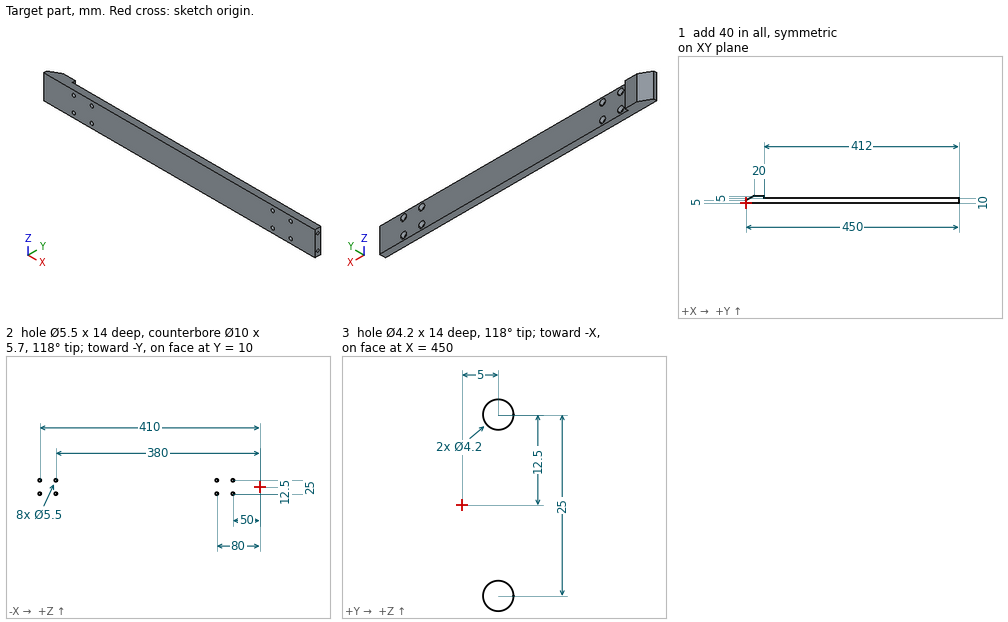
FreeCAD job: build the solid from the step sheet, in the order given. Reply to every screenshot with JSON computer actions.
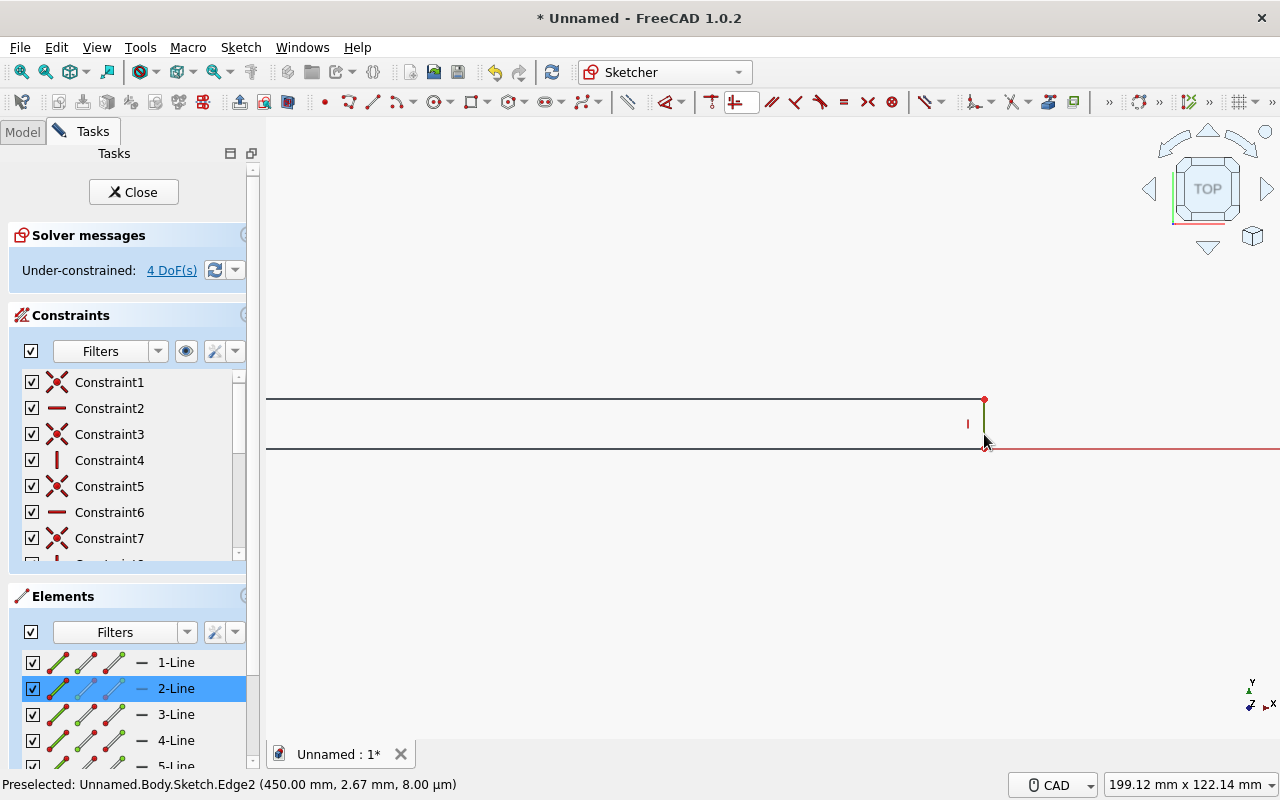
{"action": "left_click", "coordinate": [684, 102]}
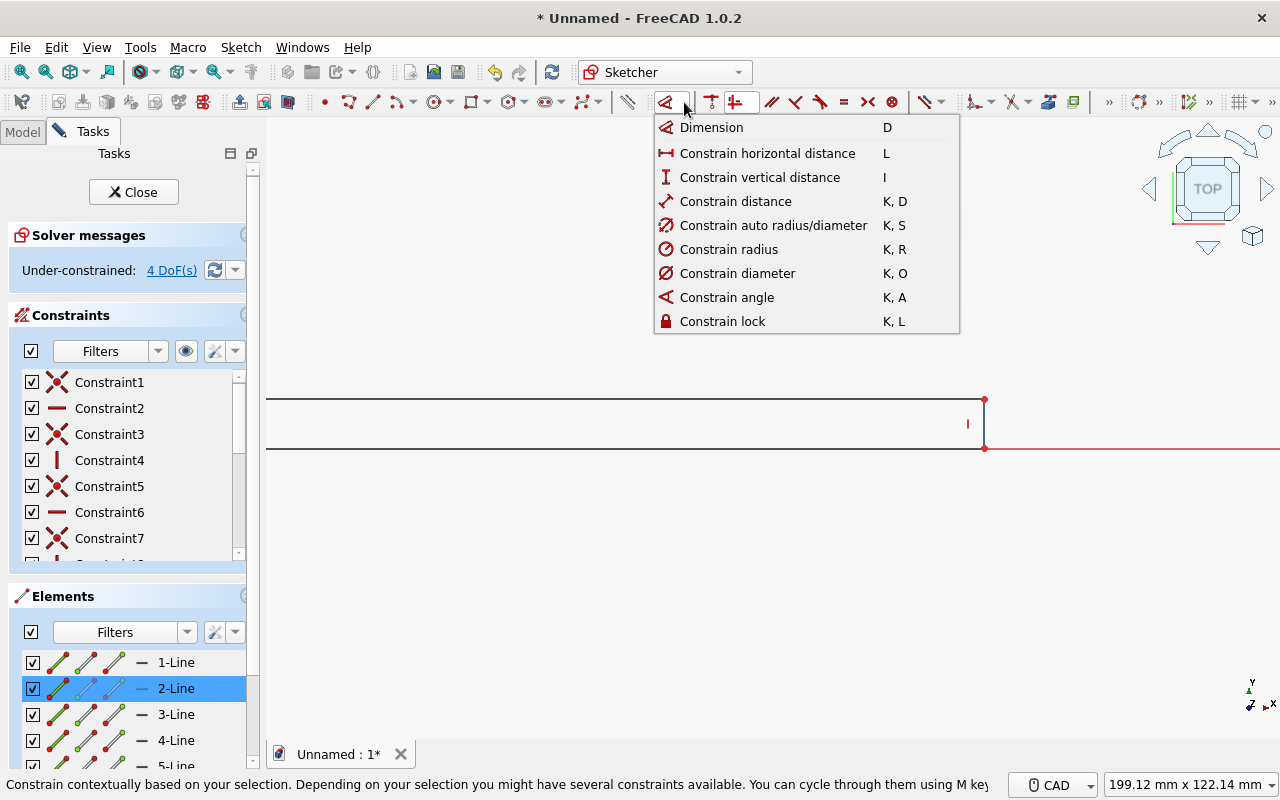
{"action": "left_click", "coordinate": [807, 177]}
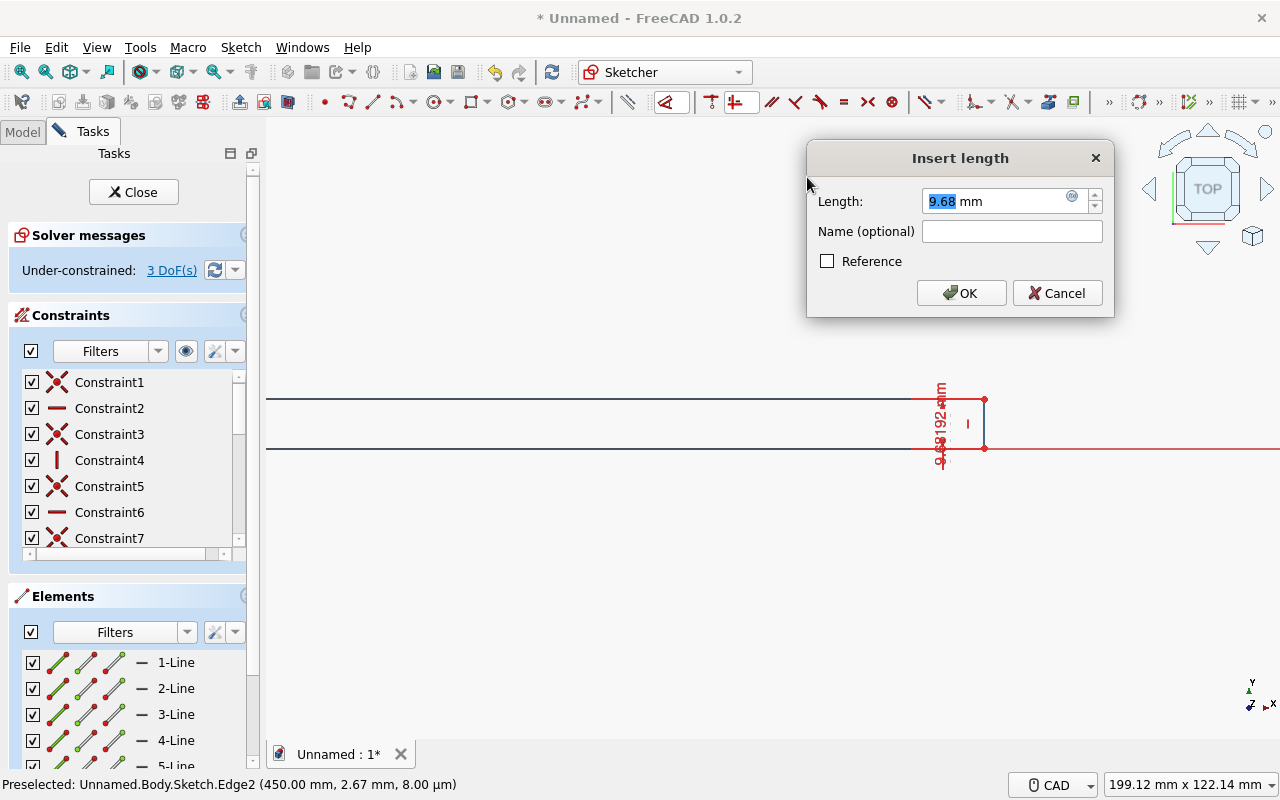
{"action": "type", "text": "10"}
{"action": "key", "text": "Return"}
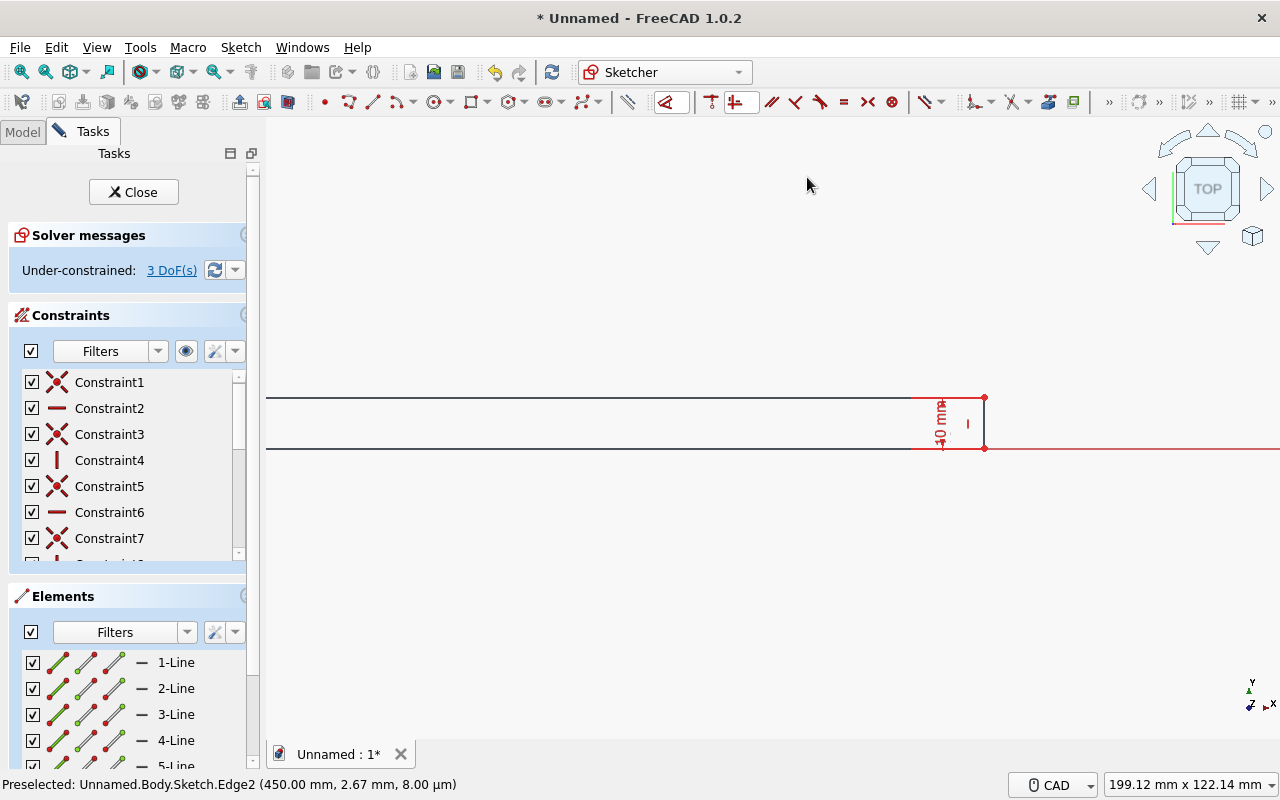
{"action": "scroll", "coordinate": [988, 434], "scroll_direction": "down", "scroll_amount": 7}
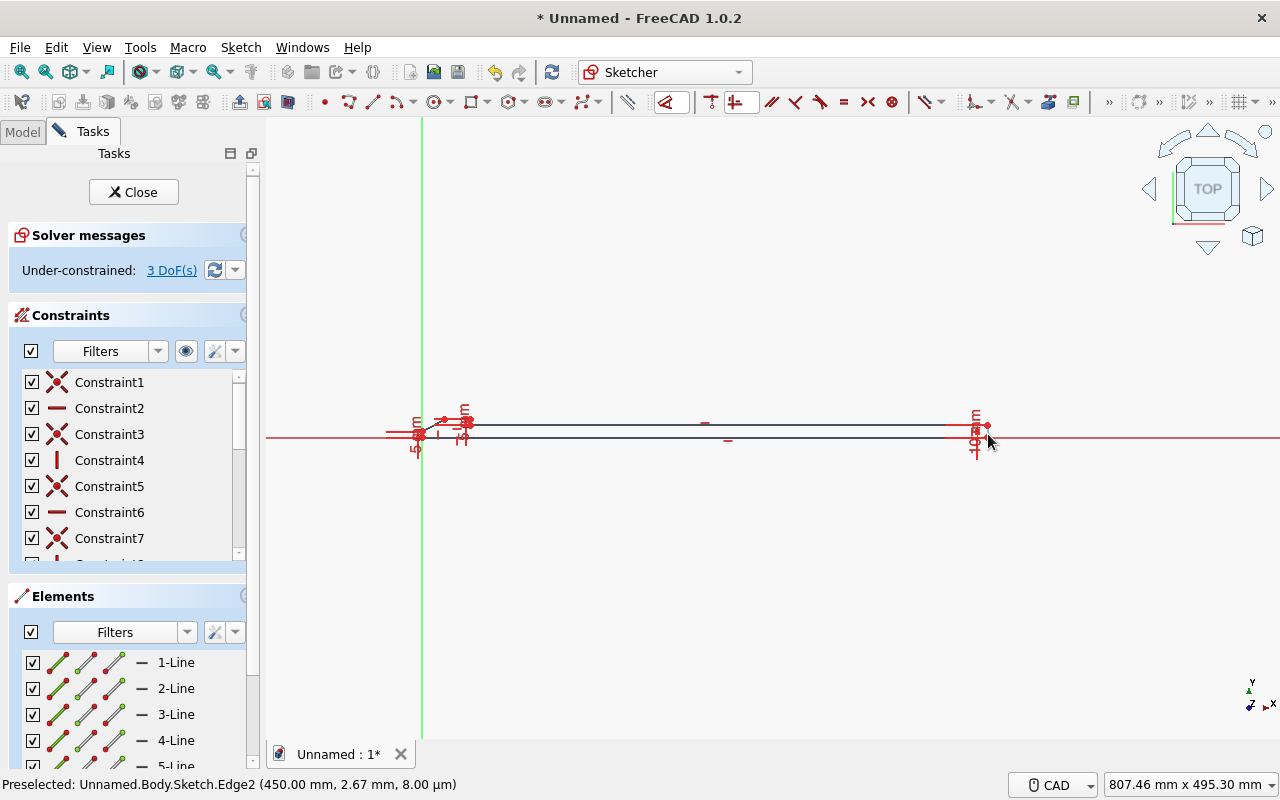
{"action": "scroll", "coordinate": [463, 419], "scroll_direction": "up", "scroll_amount": 3}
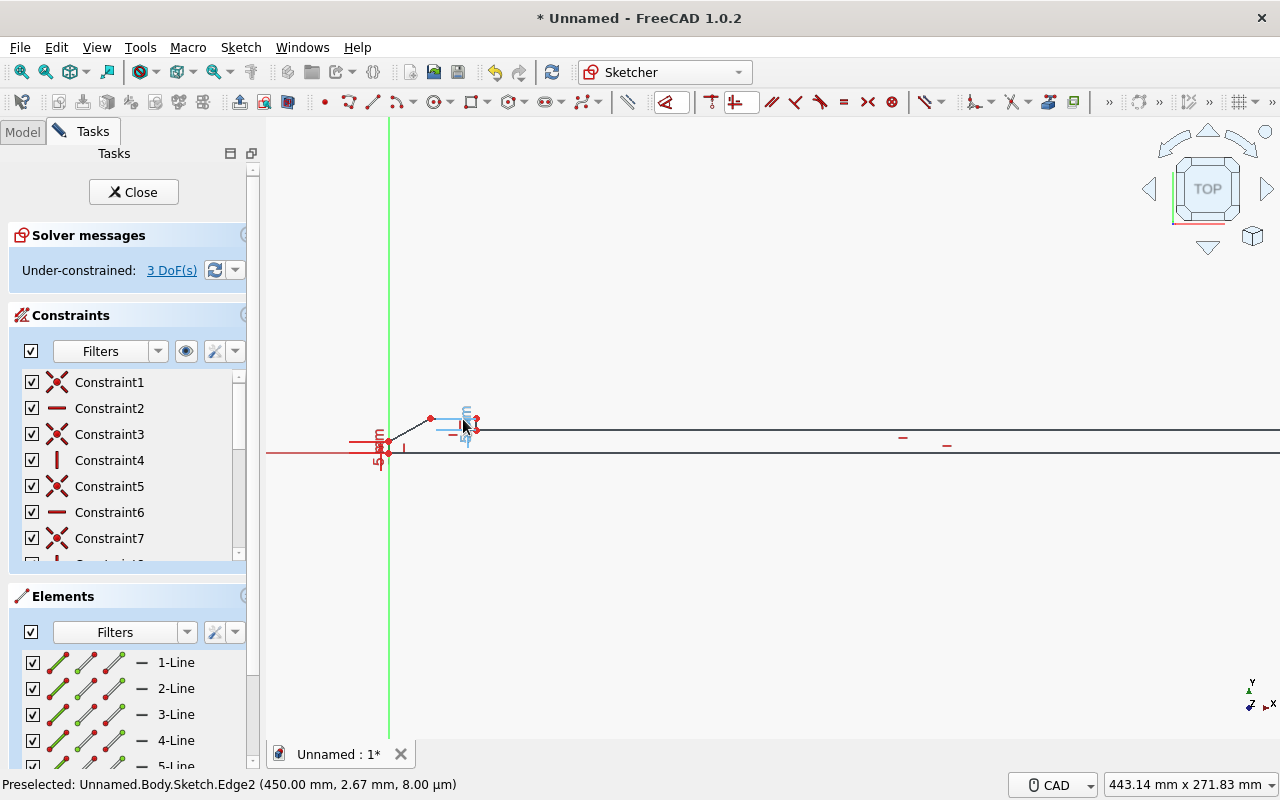
{"action": "left_click", "coordinate": [444, 419]}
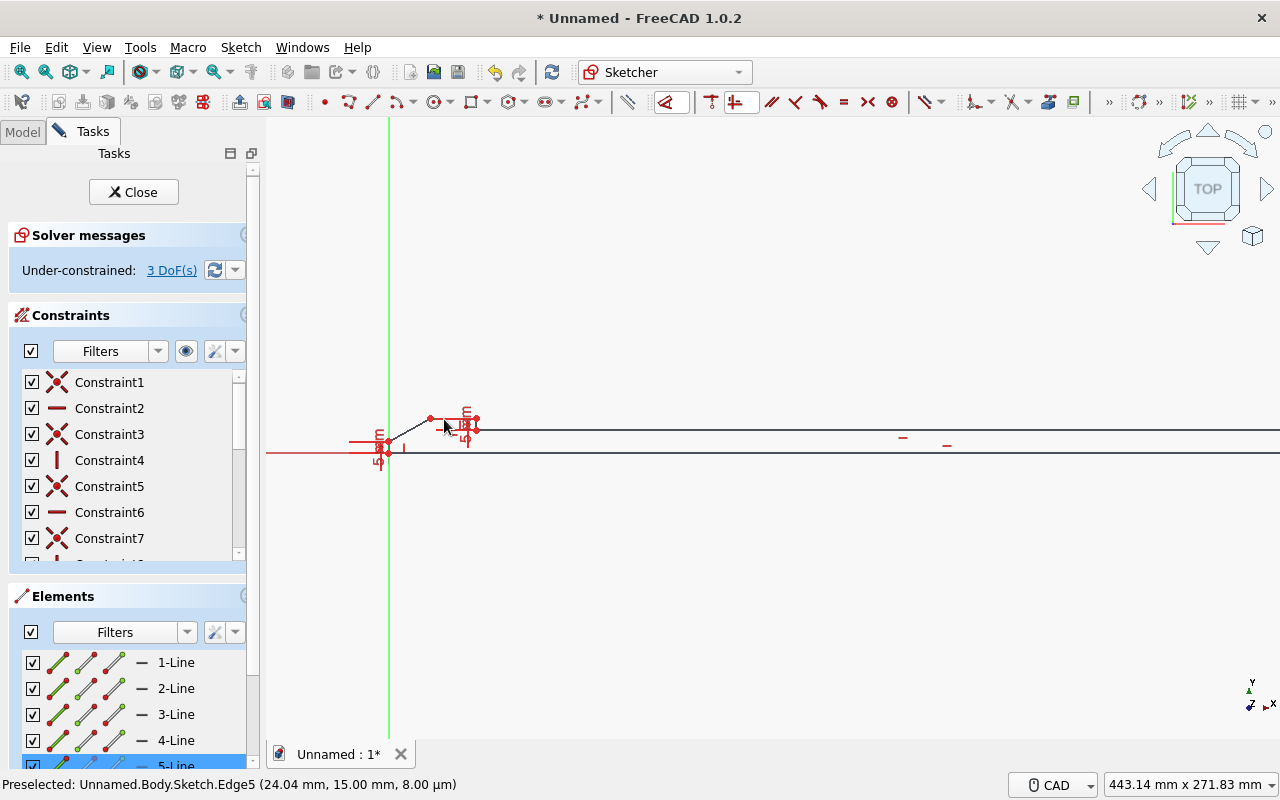
{"action": "key", "text": "l"}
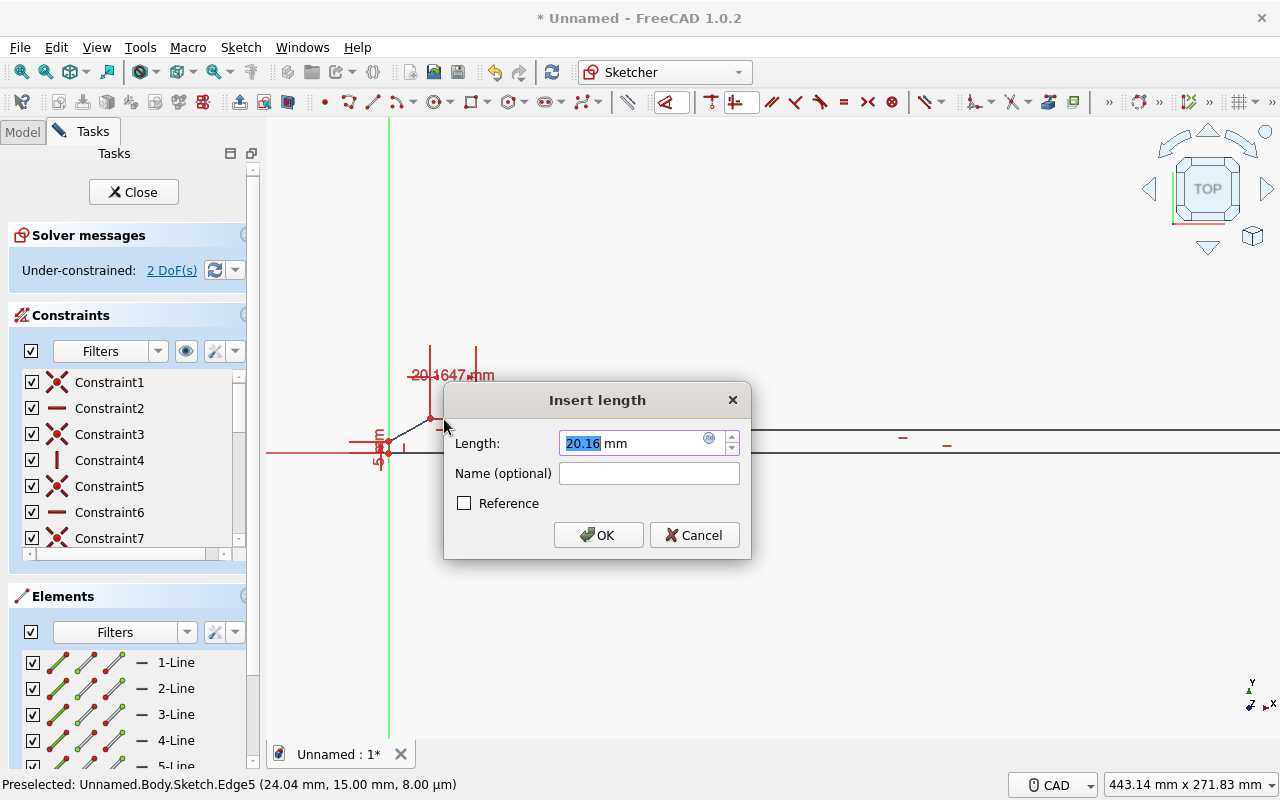
{"action": "type", "text": "20"}
{"action": "key", "text": "Return"}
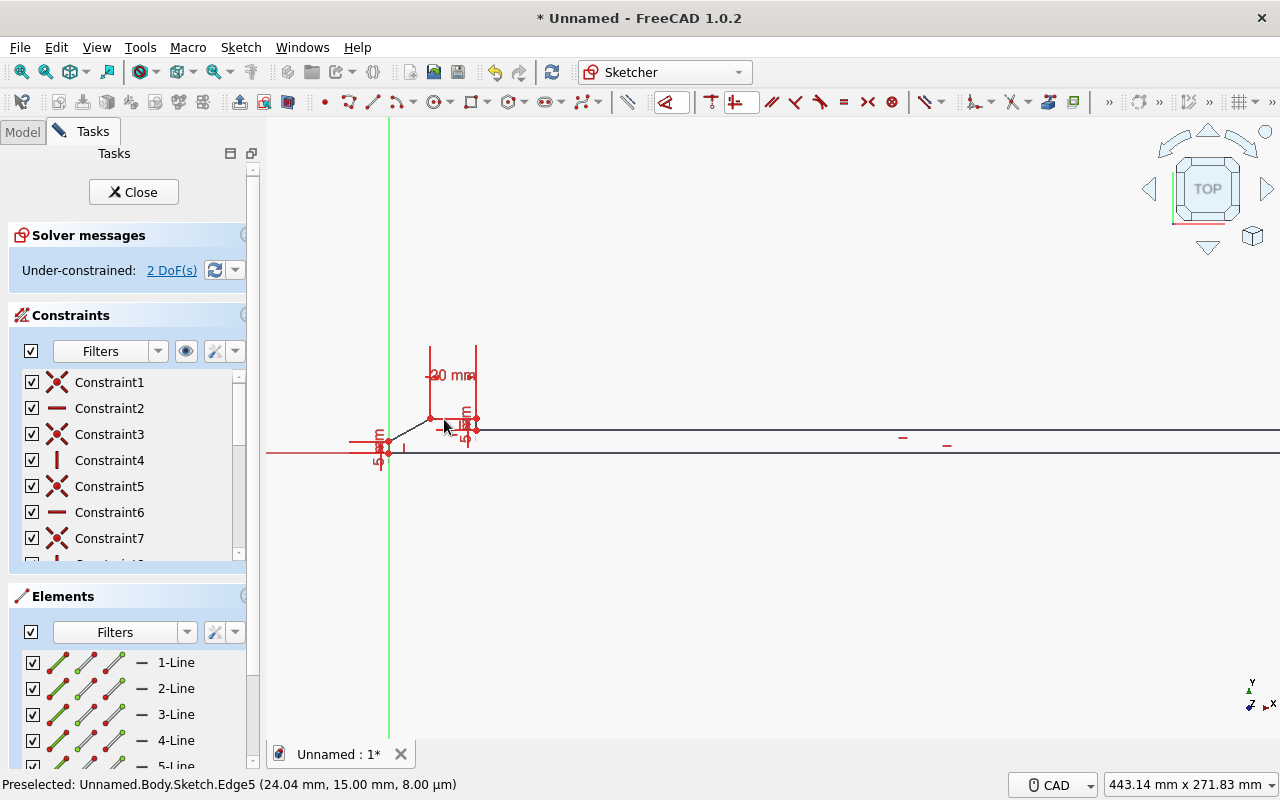
{"action": "left_click", "coordinate": [698, 453]}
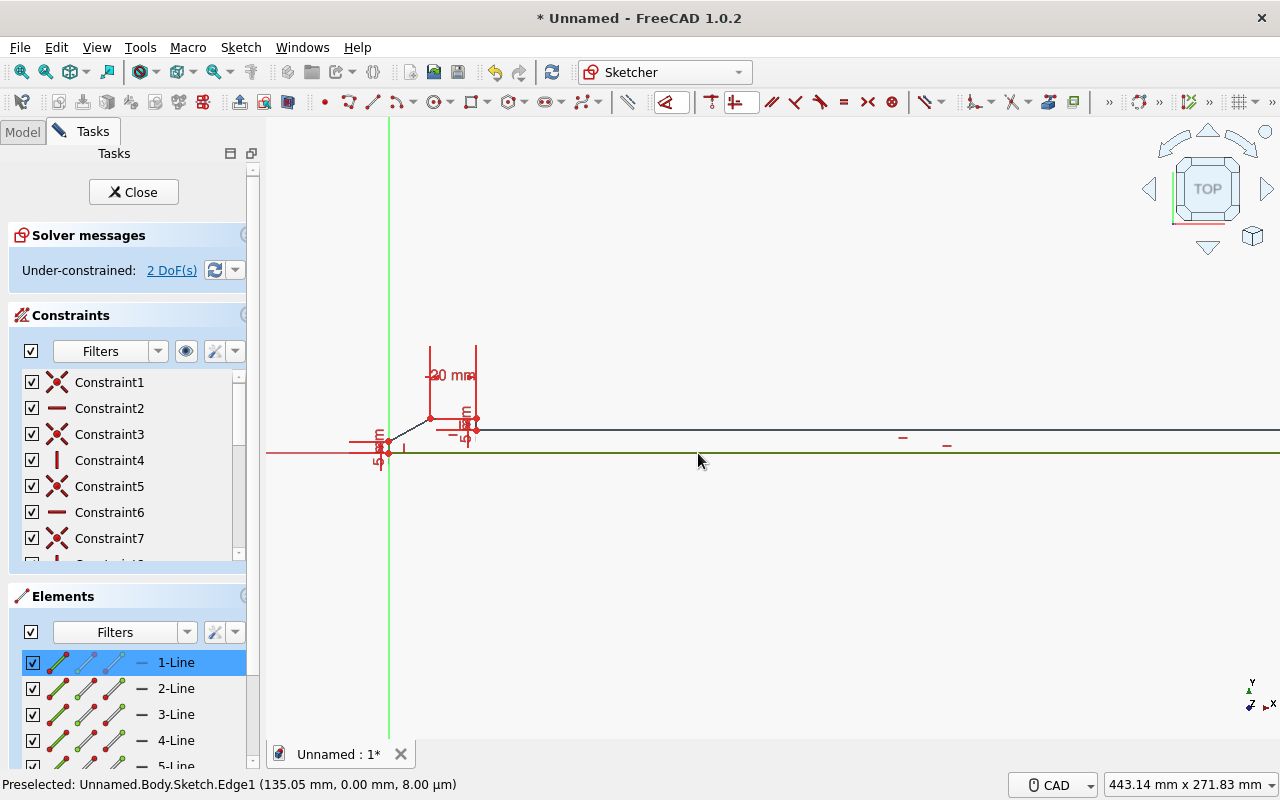
{"action": "left_click", "coordinate": [684, 102]}